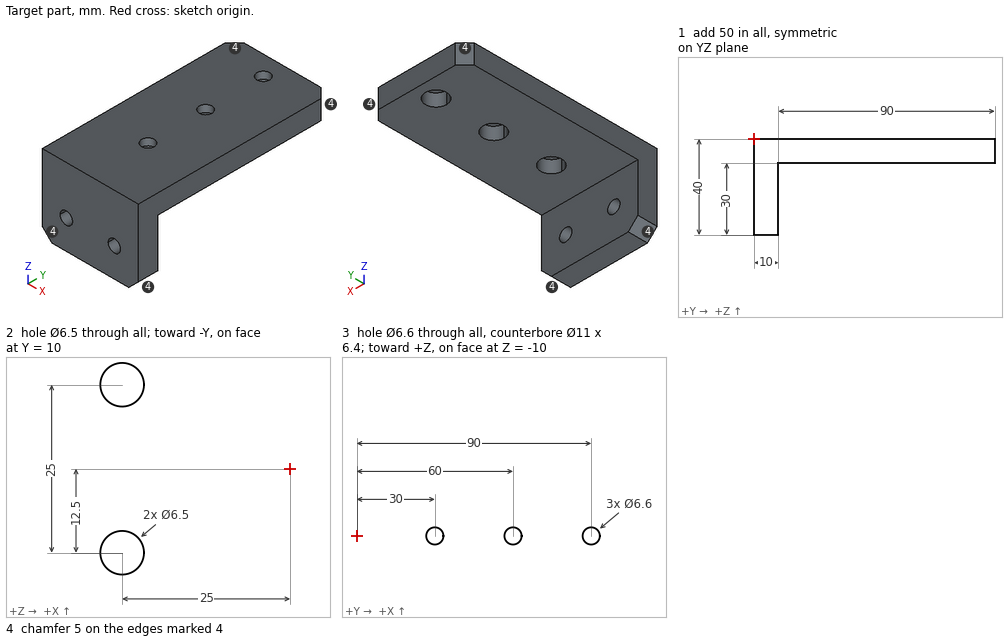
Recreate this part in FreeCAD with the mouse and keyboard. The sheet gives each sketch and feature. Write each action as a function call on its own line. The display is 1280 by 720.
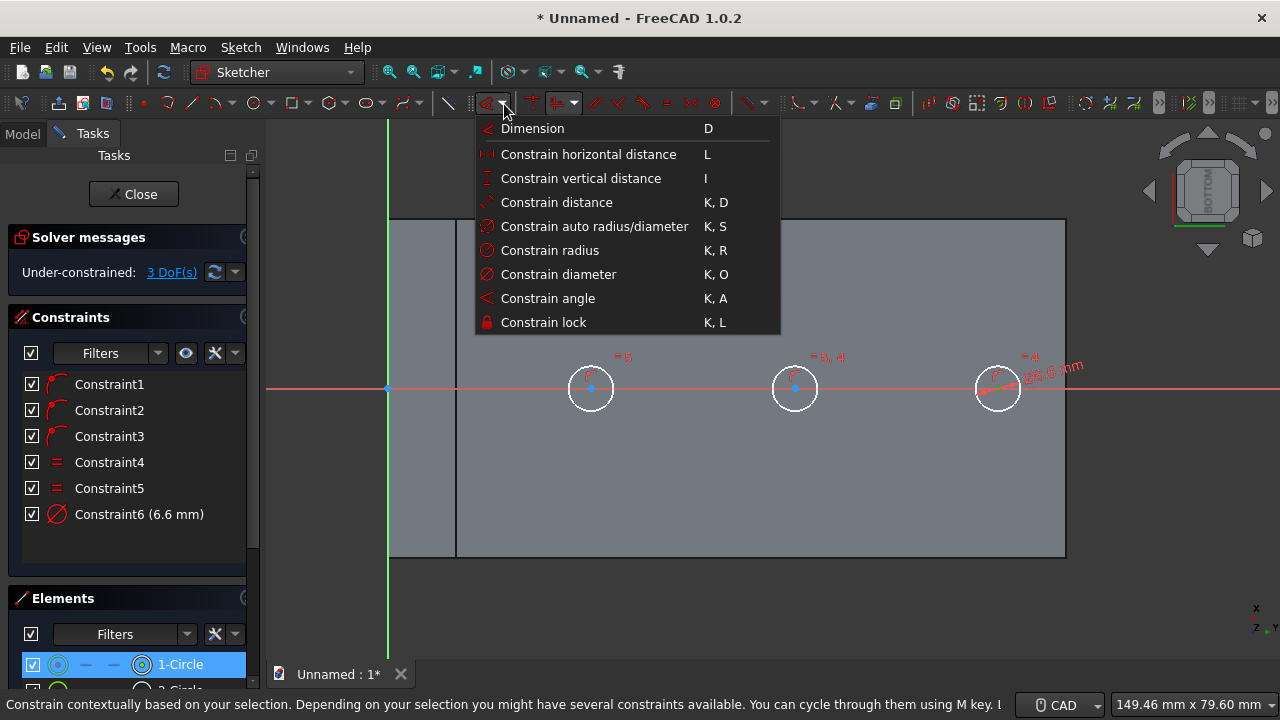
click(628, 154)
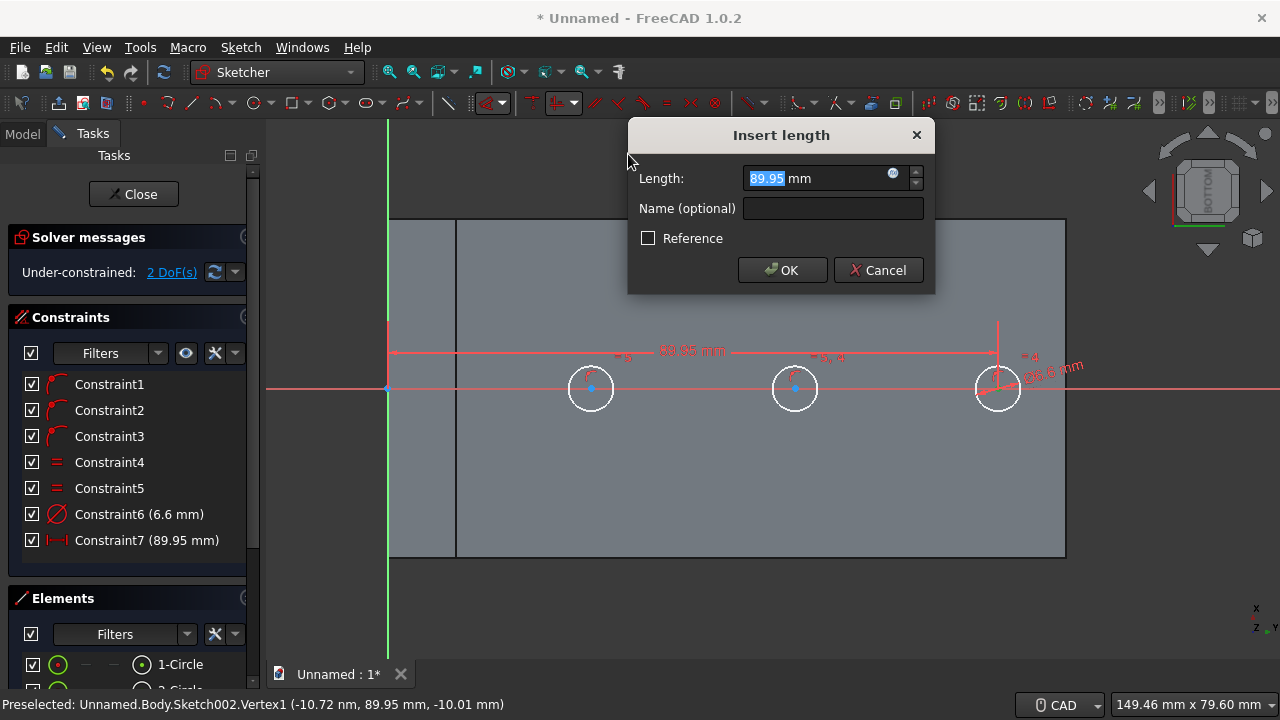
text(90)
key(Return)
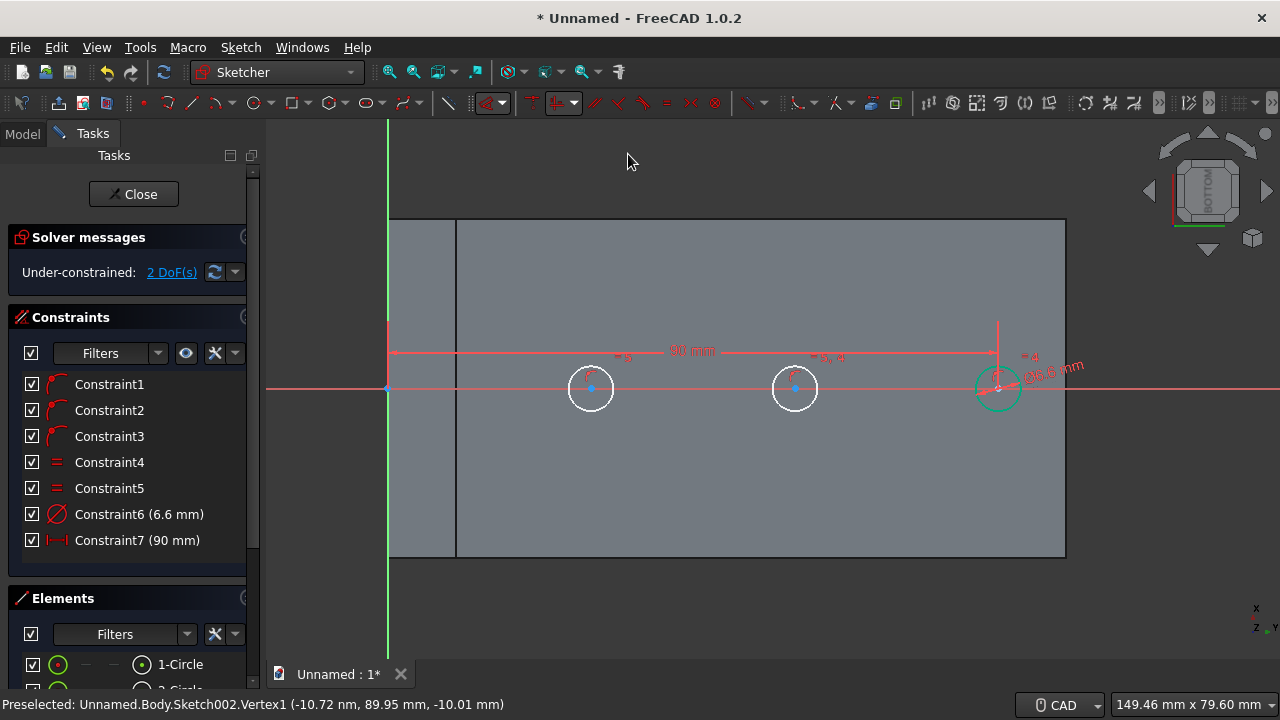
click(795, 389)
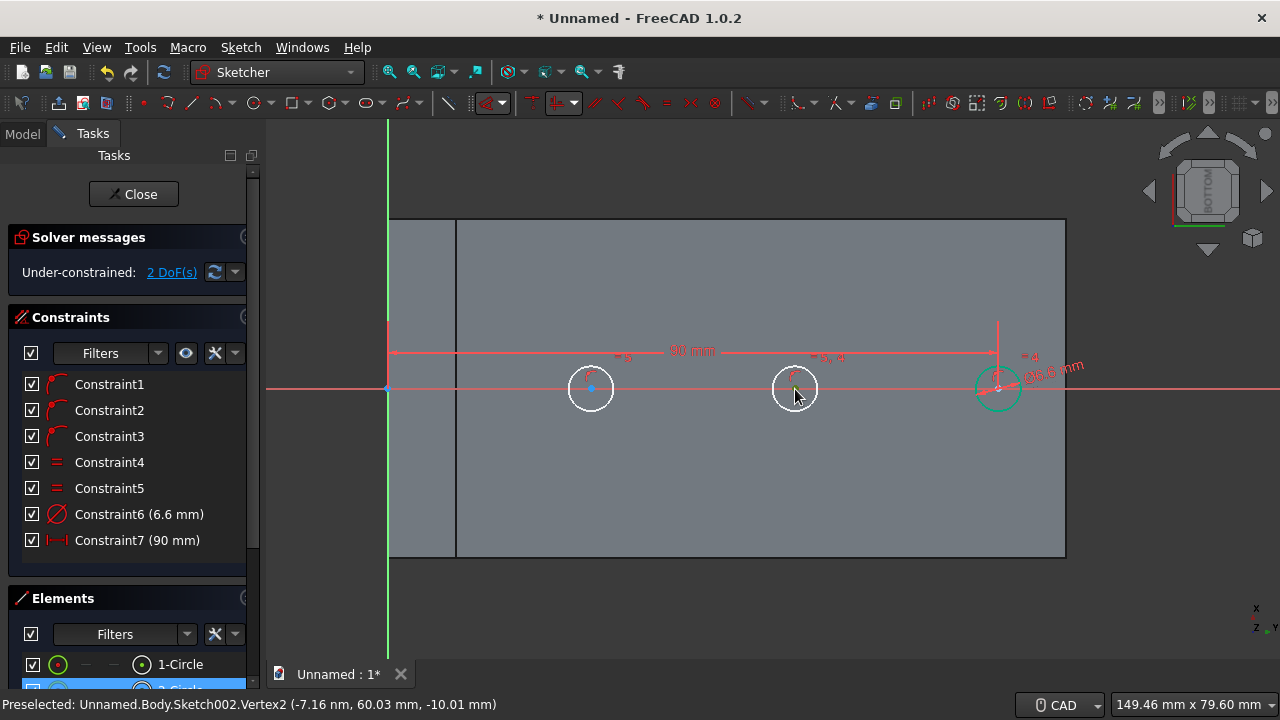
click(504, 104)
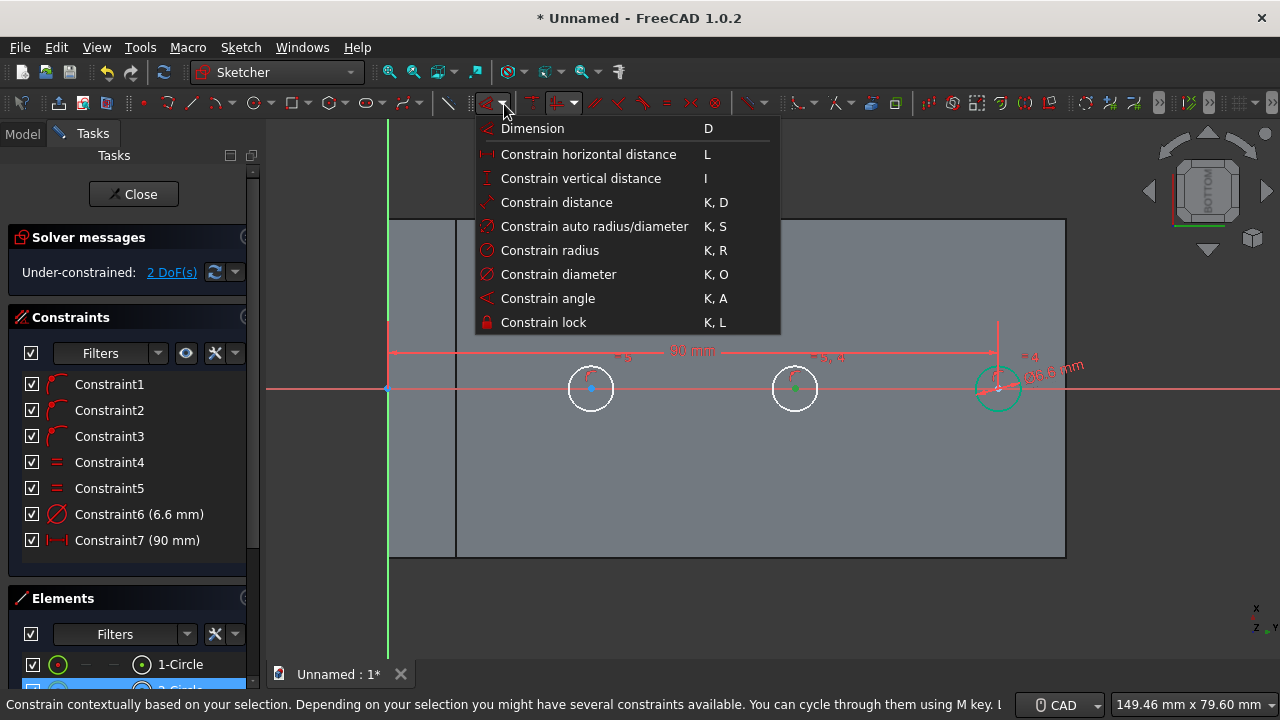
click(628, 154)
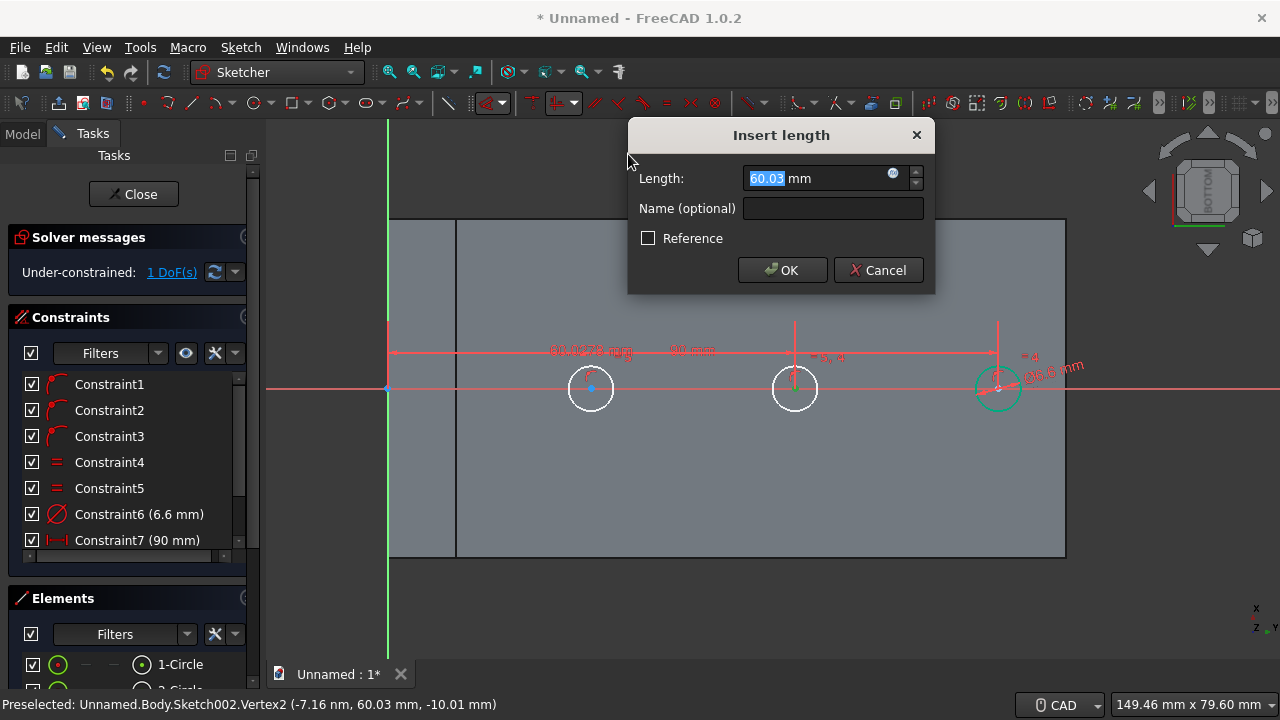
text(60)
key(Return)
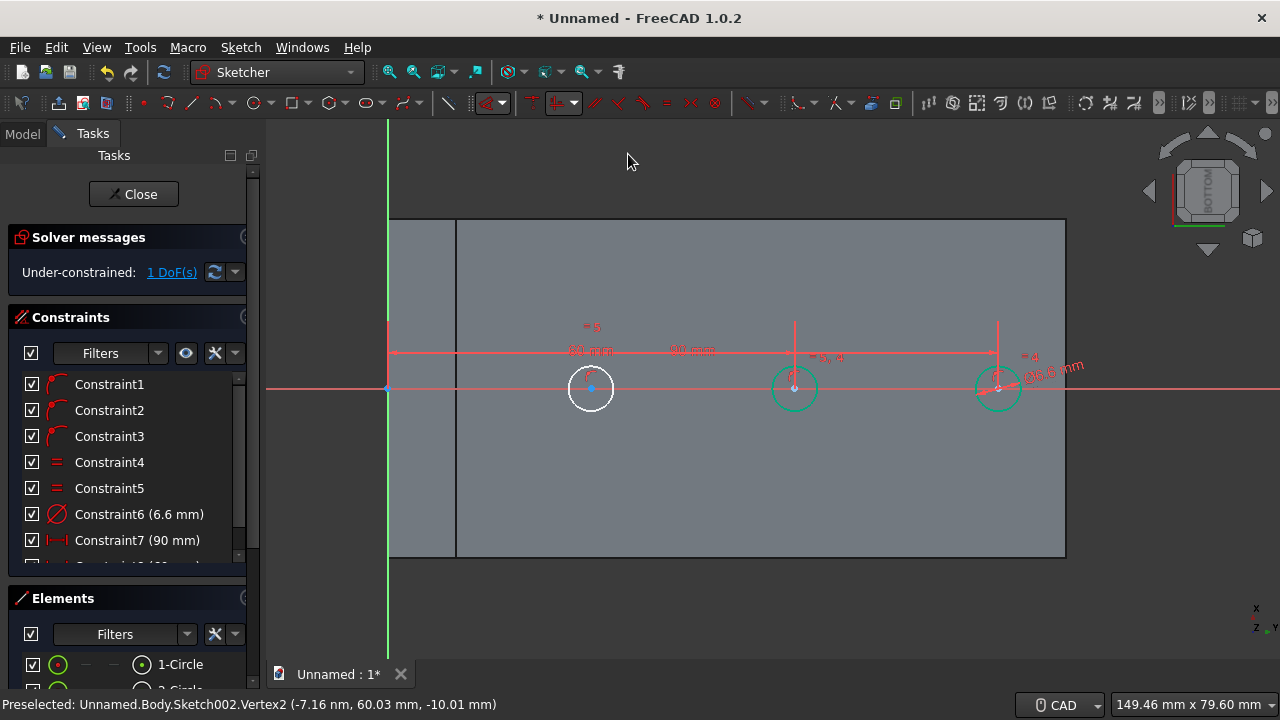
click(591, 389)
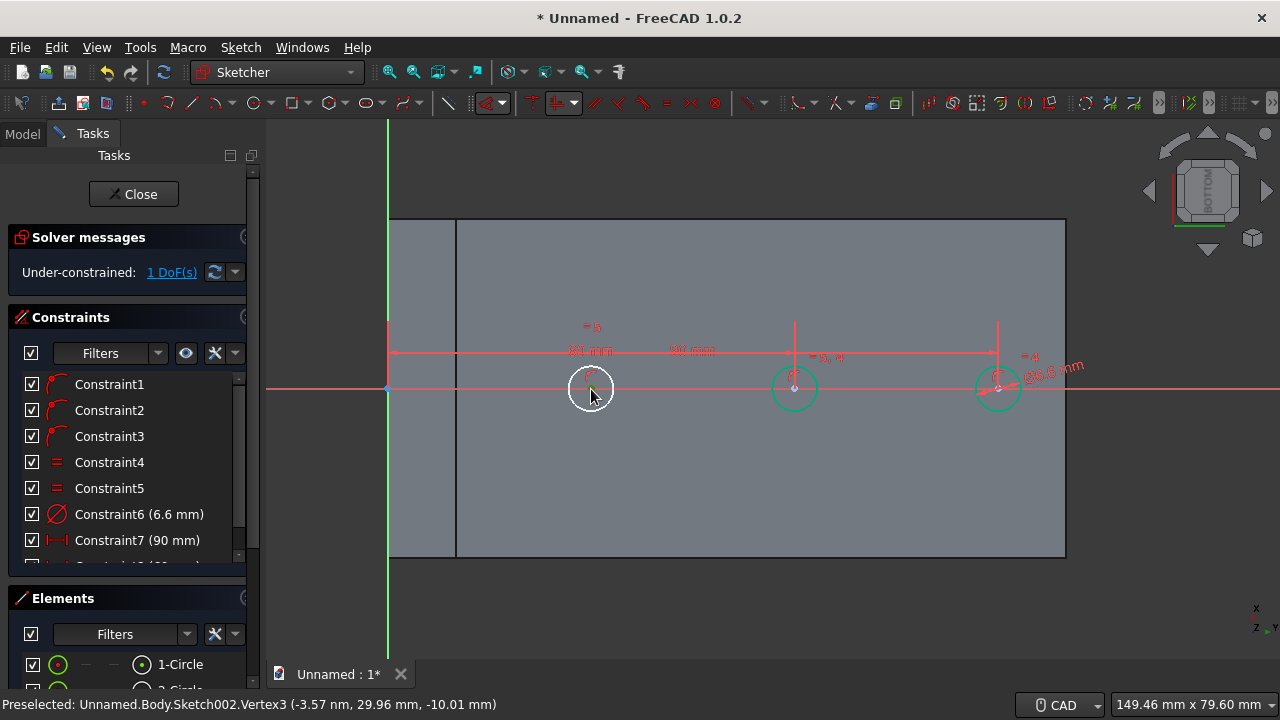
key(l)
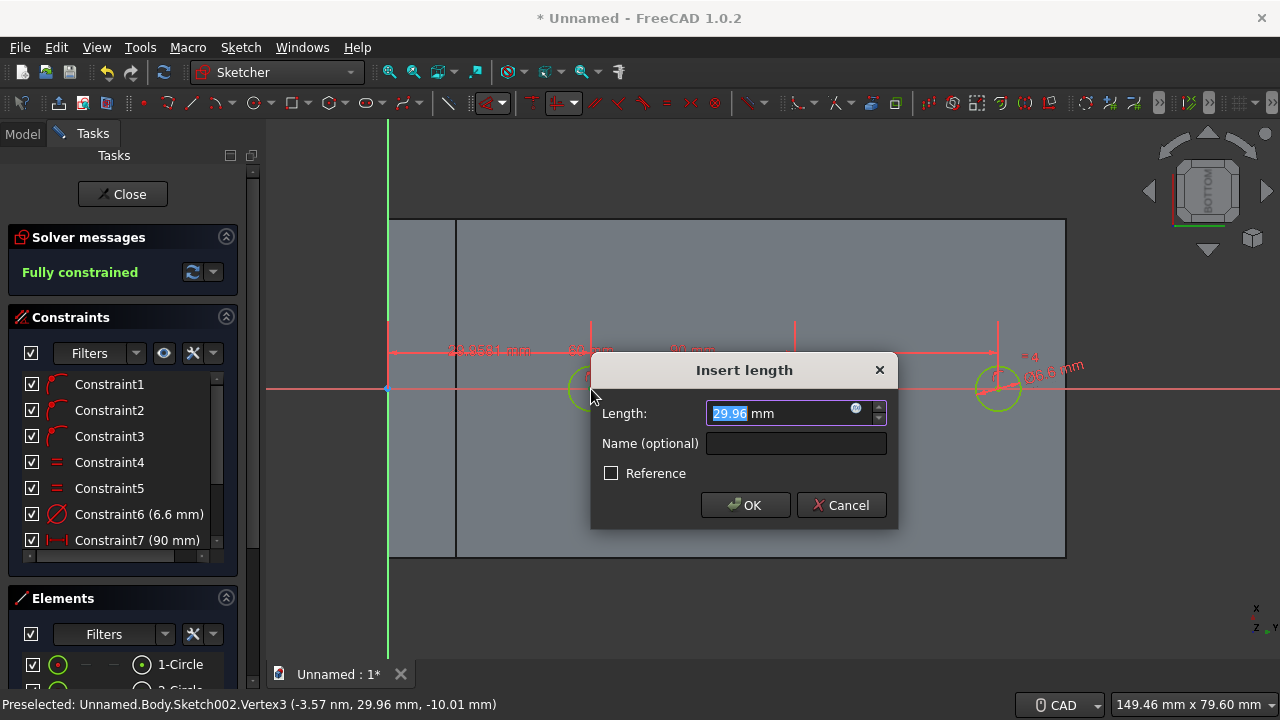
text(30)
key(Return)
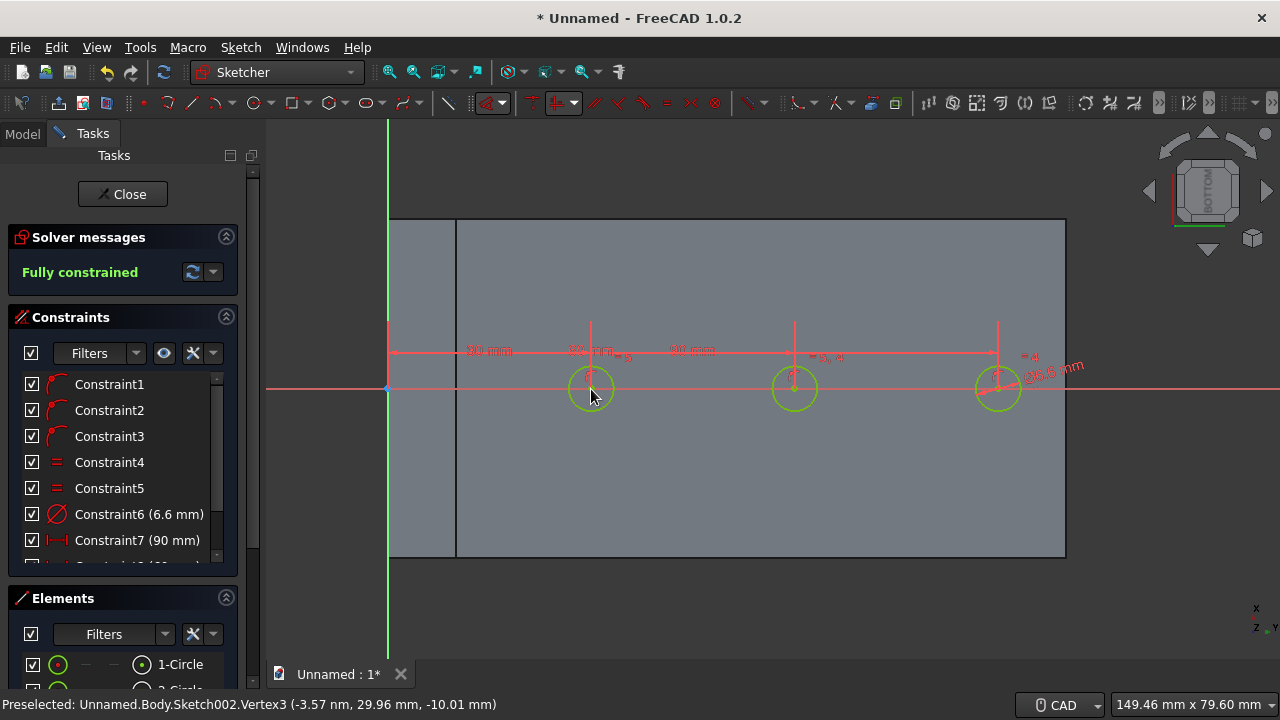
click(123, 194)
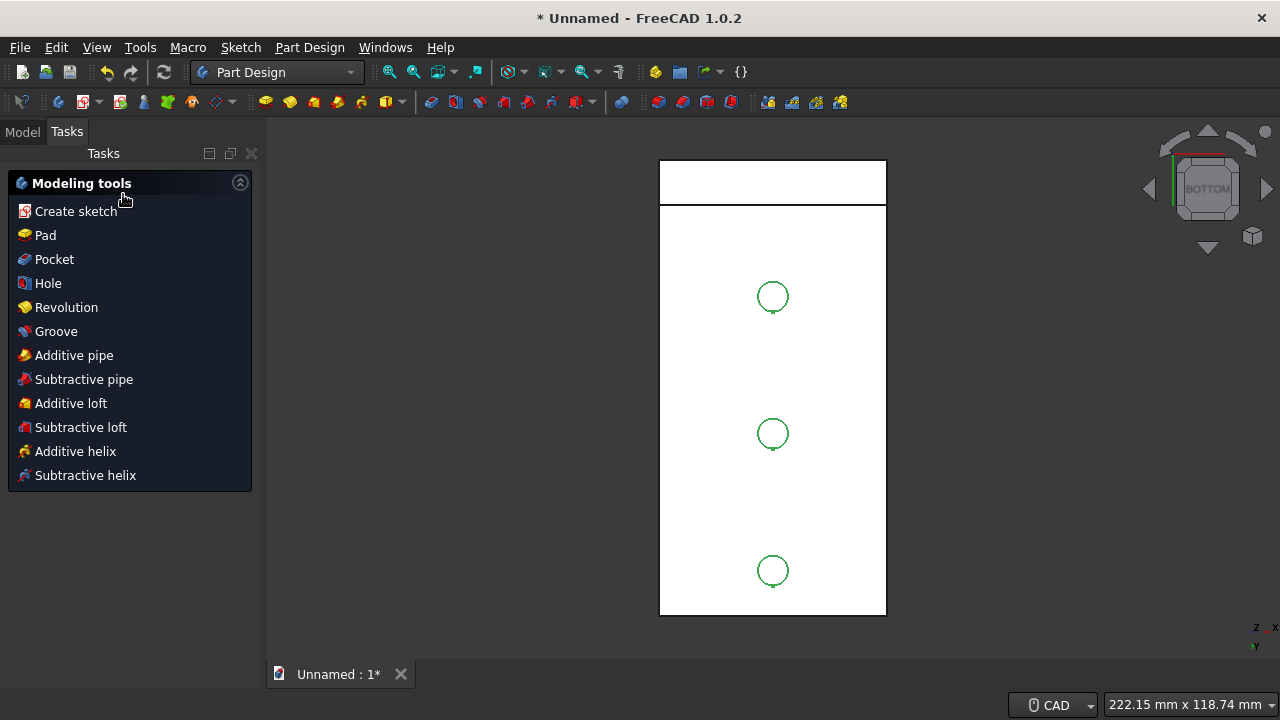
click(456, 102)